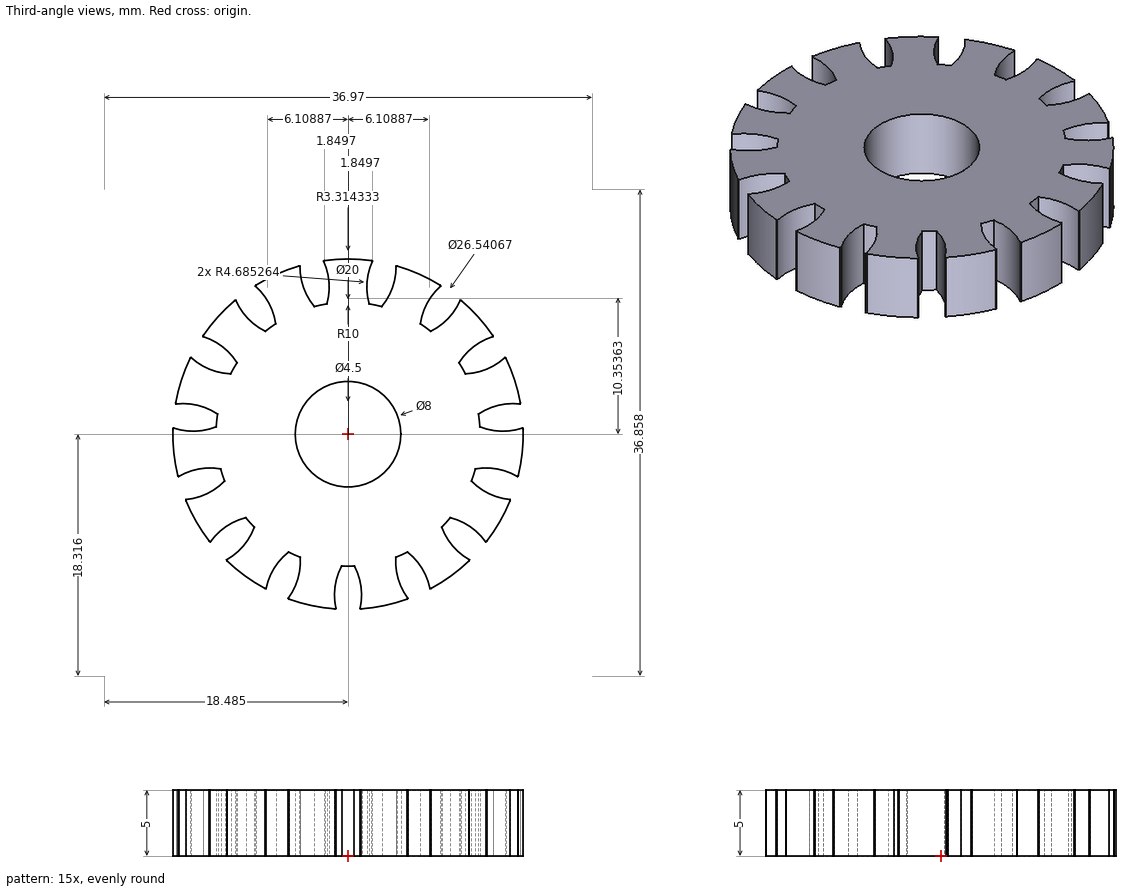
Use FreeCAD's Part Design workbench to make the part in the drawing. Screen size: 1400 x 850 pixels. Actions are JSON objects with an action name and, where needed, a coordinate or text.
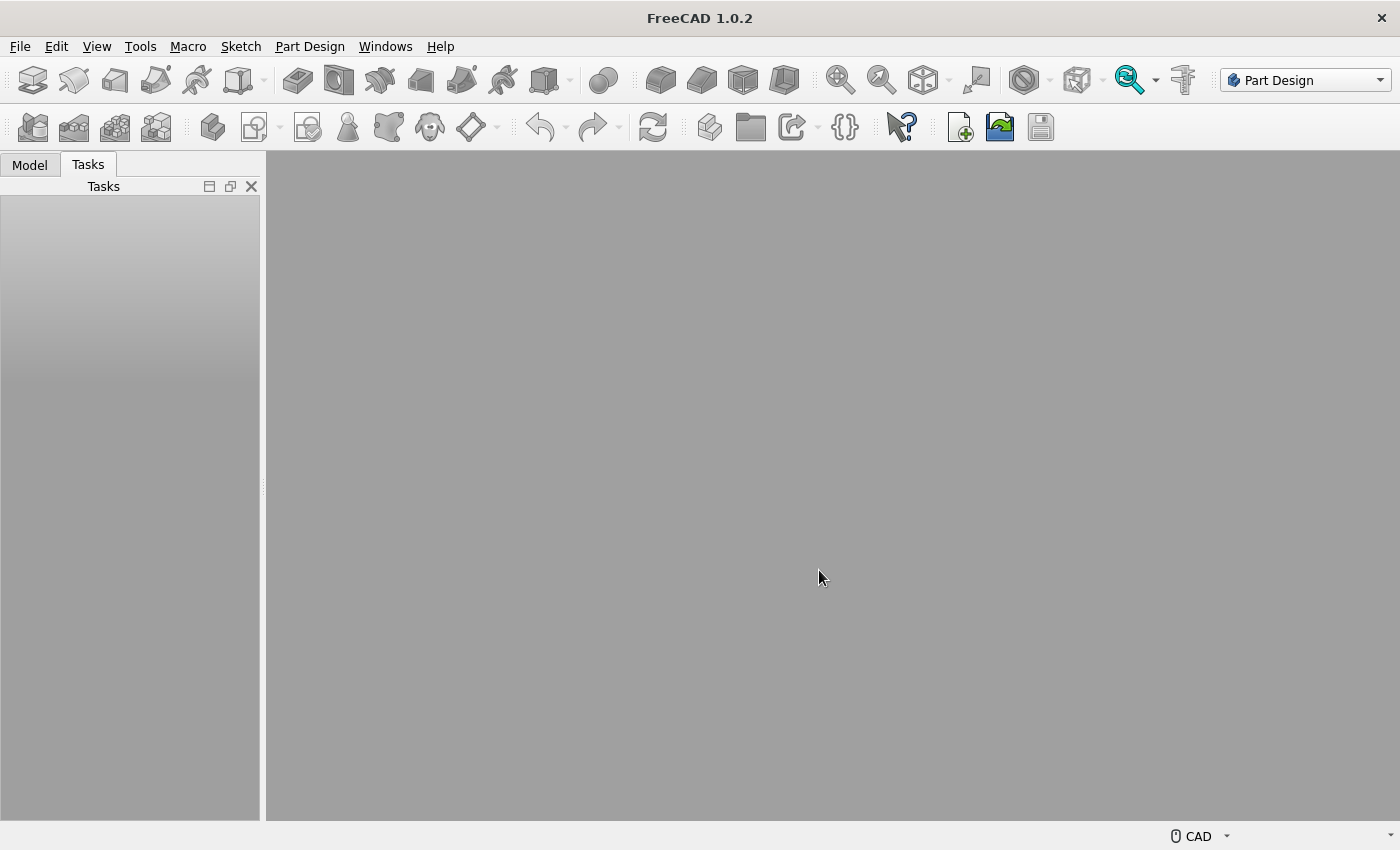
{"action": "left_click", "coordinate": [959, 128]}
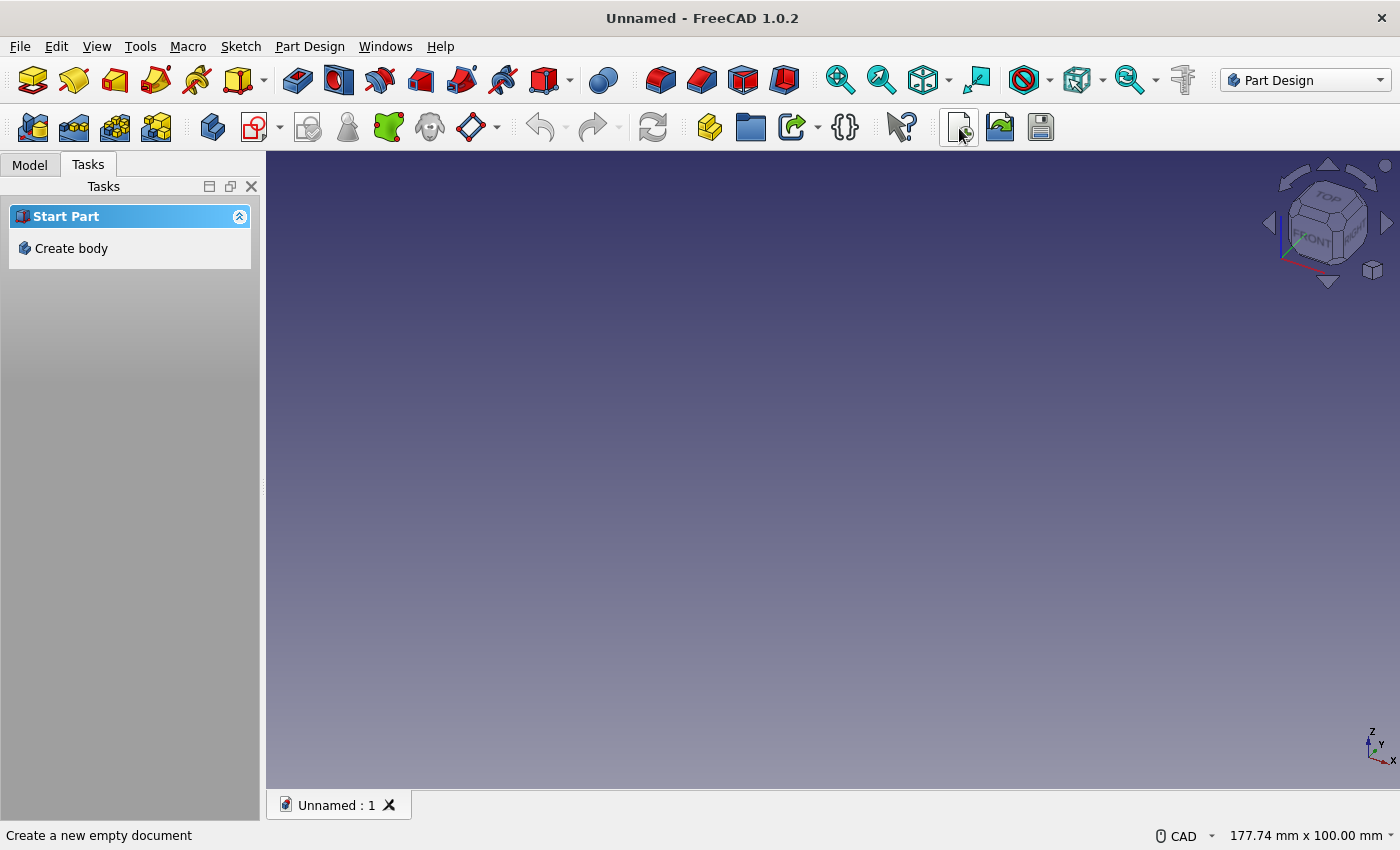
{"action": "left_click", "coordinate": [254, 128]}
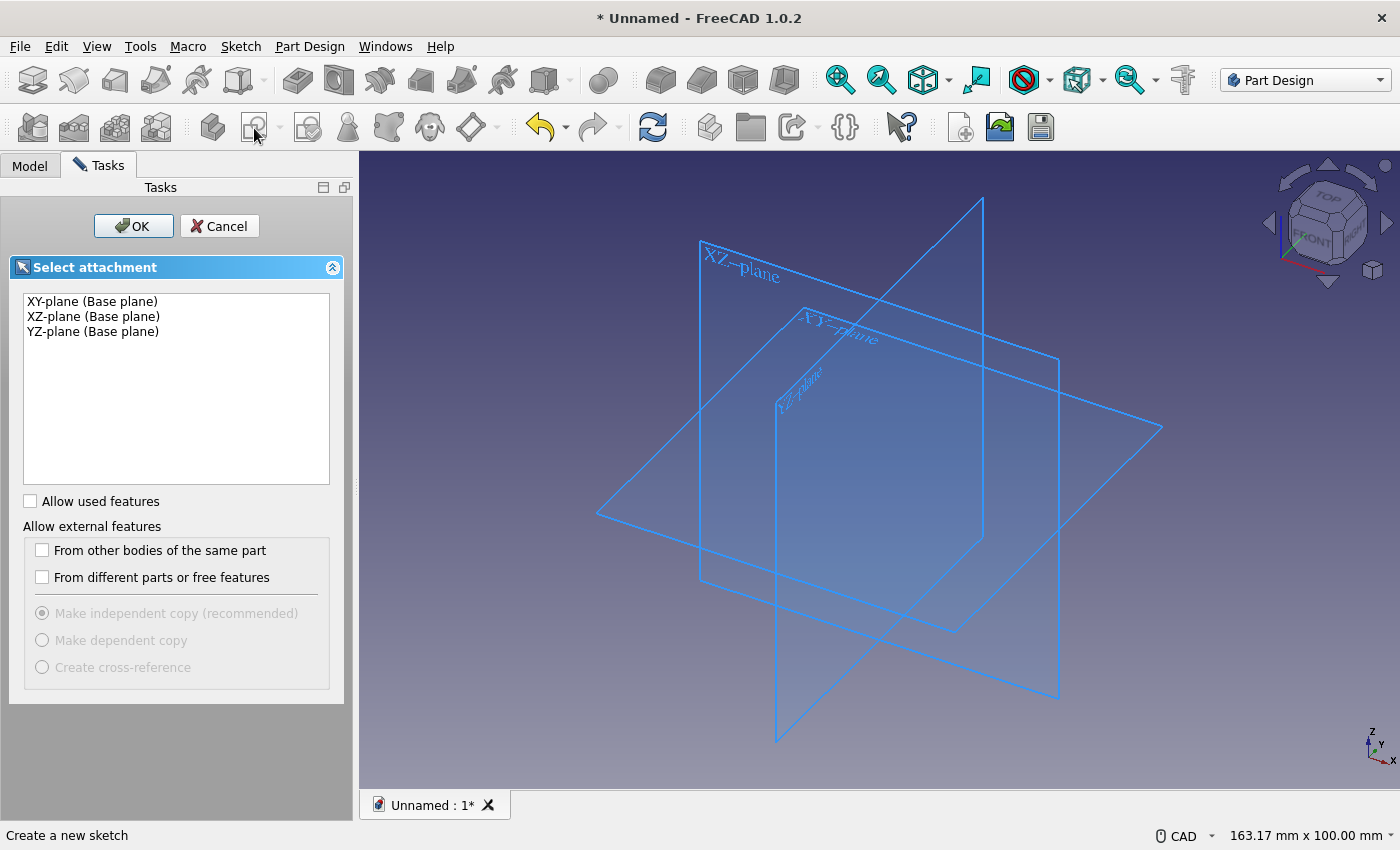
{"action": "left_click", "coordinate": [84, 302]}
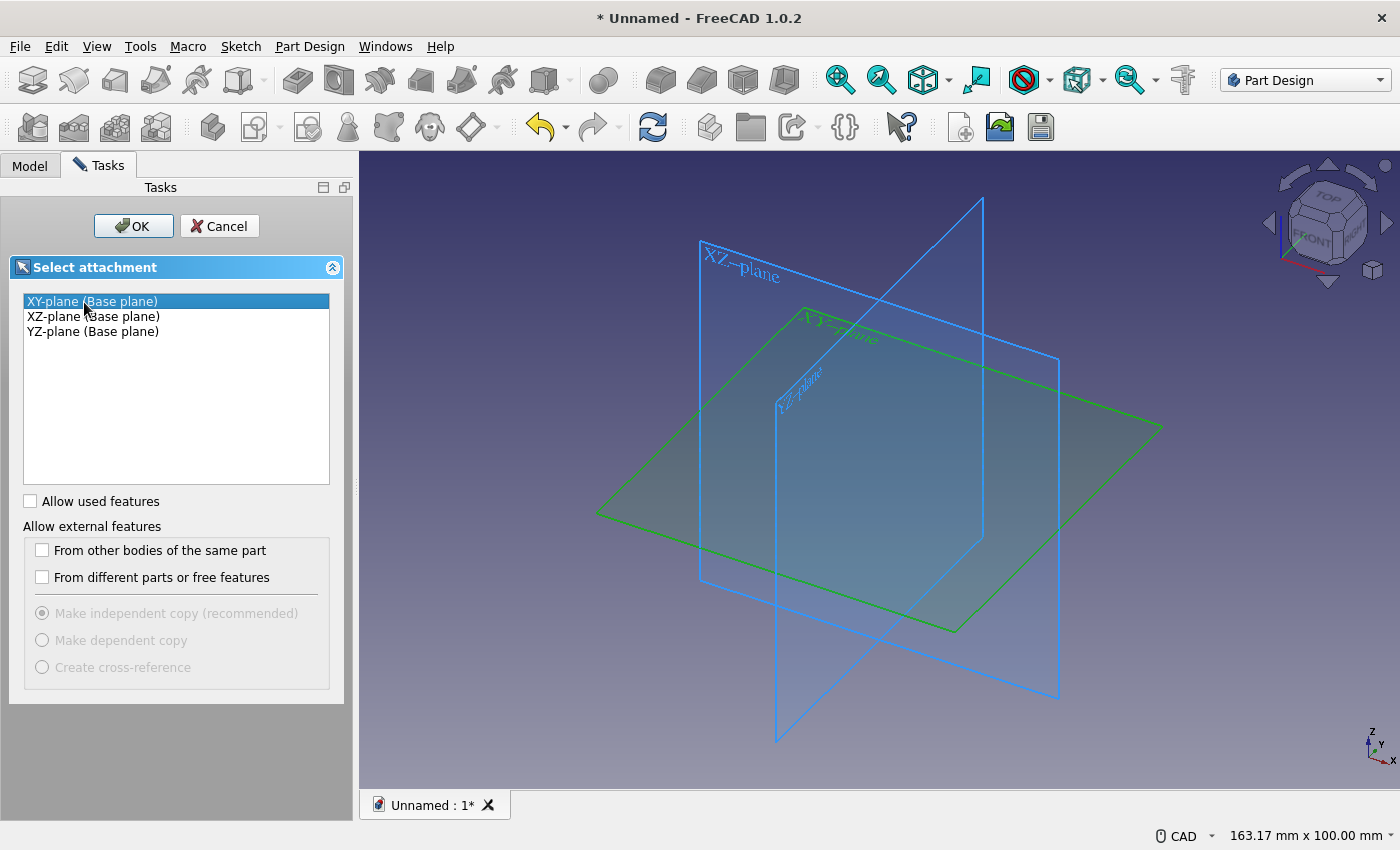
{"action": "left_click", "coordinate": [134, 226]}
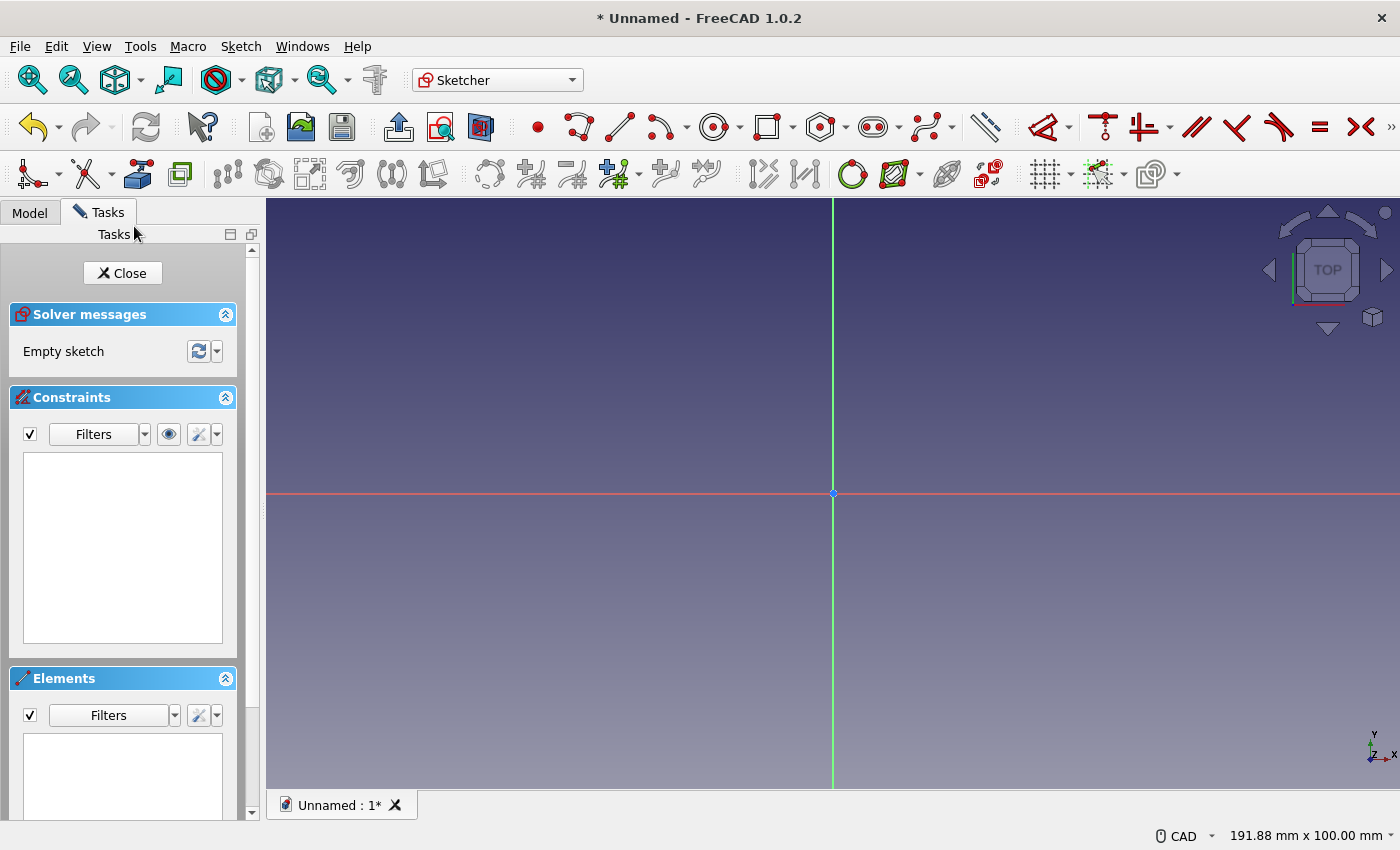
{"action": "scroll", "coordinate": [863, 494], "scroll_direction": "up", "scroll_amount": 6}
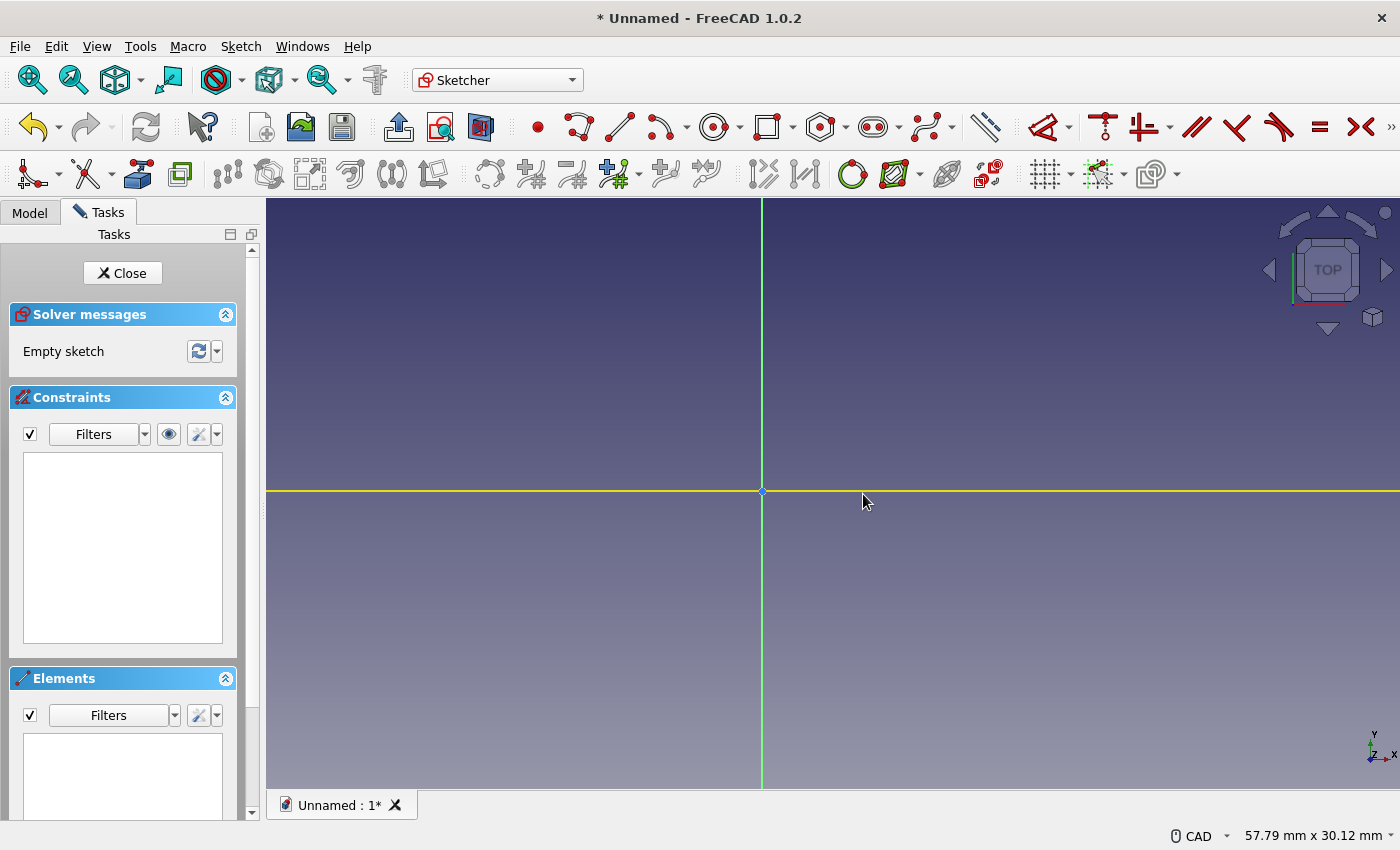
{"action": "left_click", "coordinate": [714, 128]}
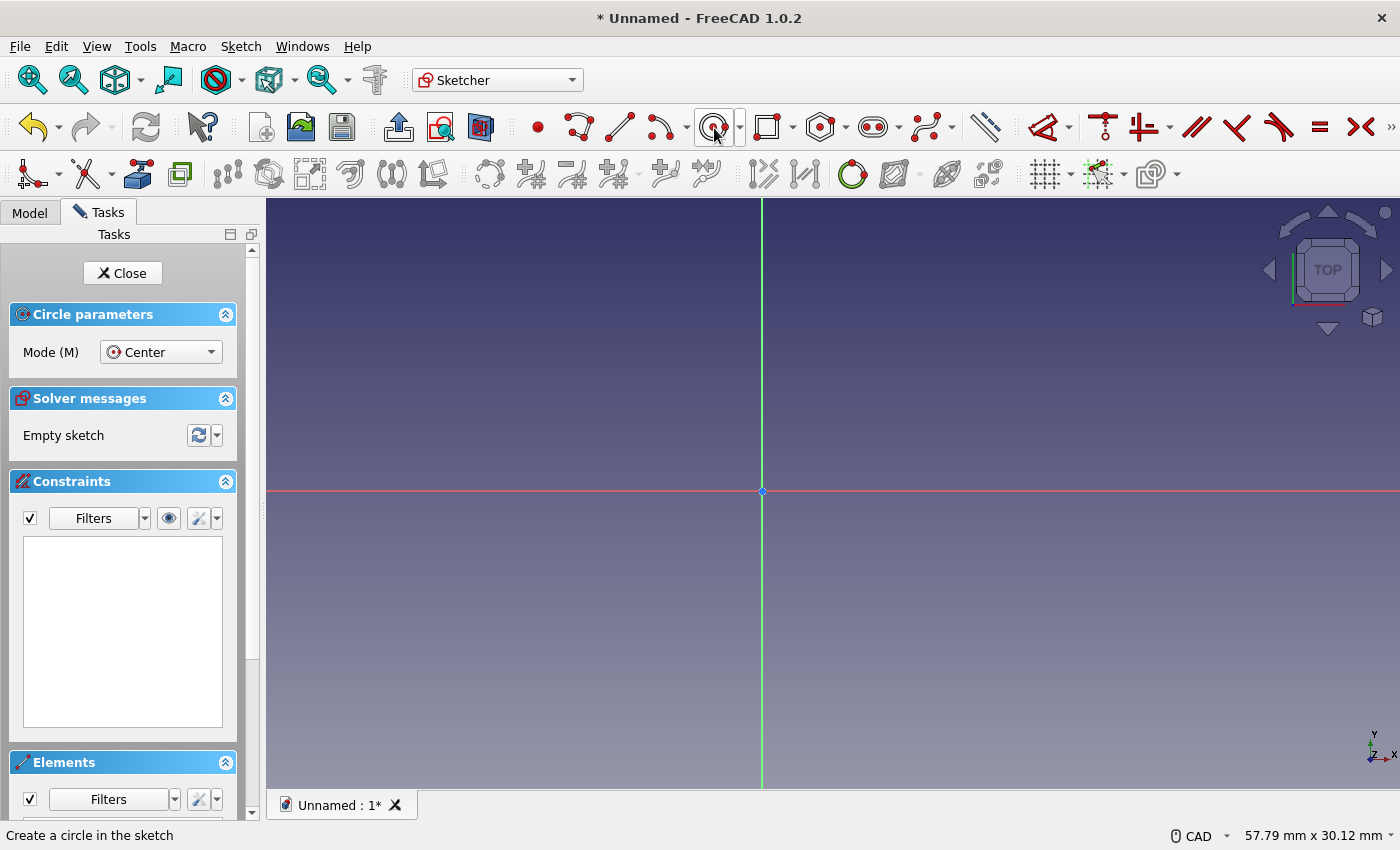
{"action": "left_click", "coordinate": [762, 491]}
{"action": "mouse_move", "coordinate": [901, 352]}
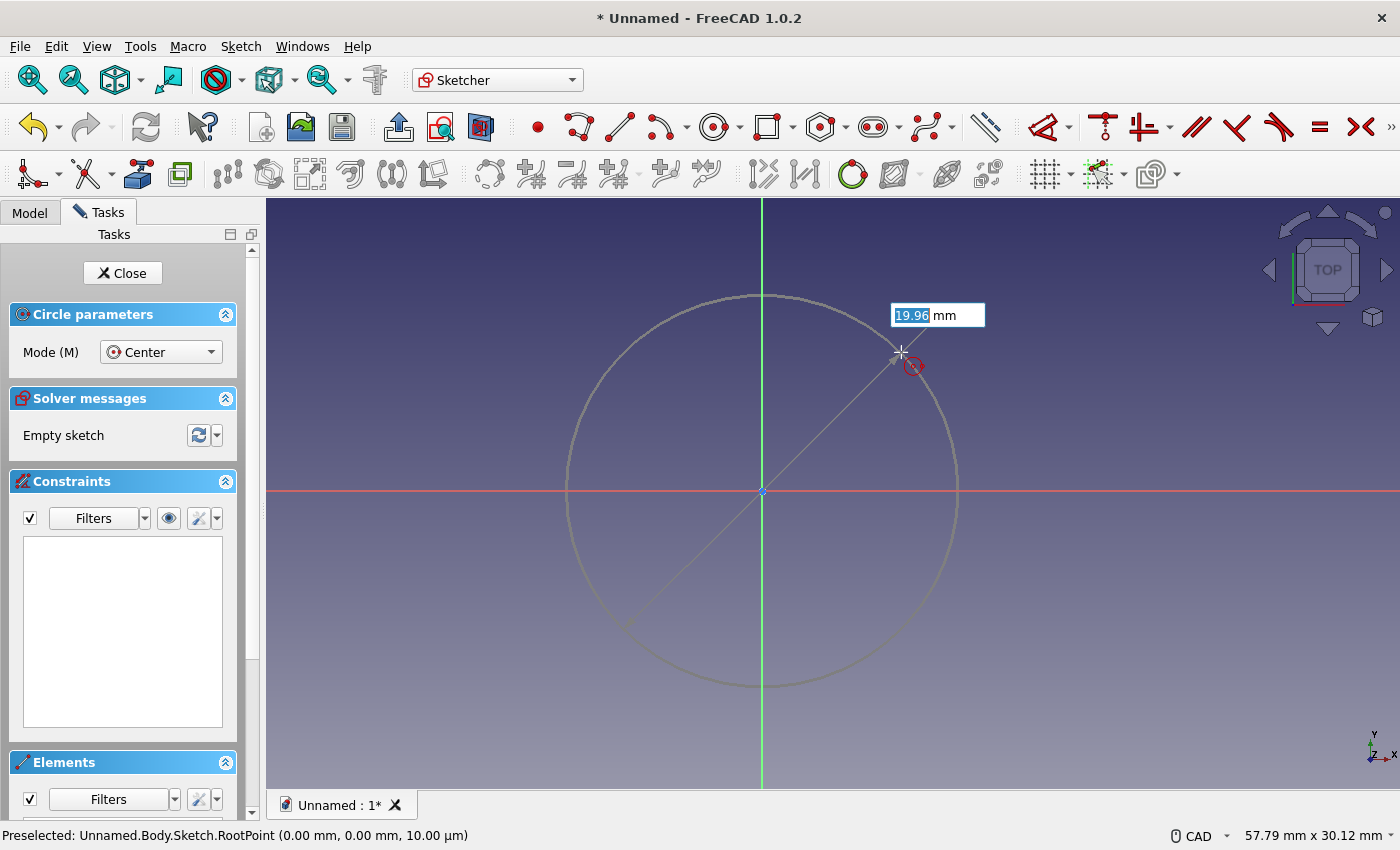
{"action": "type", "text": "20"}
{"action": "key", "text": "Return"}
{"action": "key", "text": "Escape"}